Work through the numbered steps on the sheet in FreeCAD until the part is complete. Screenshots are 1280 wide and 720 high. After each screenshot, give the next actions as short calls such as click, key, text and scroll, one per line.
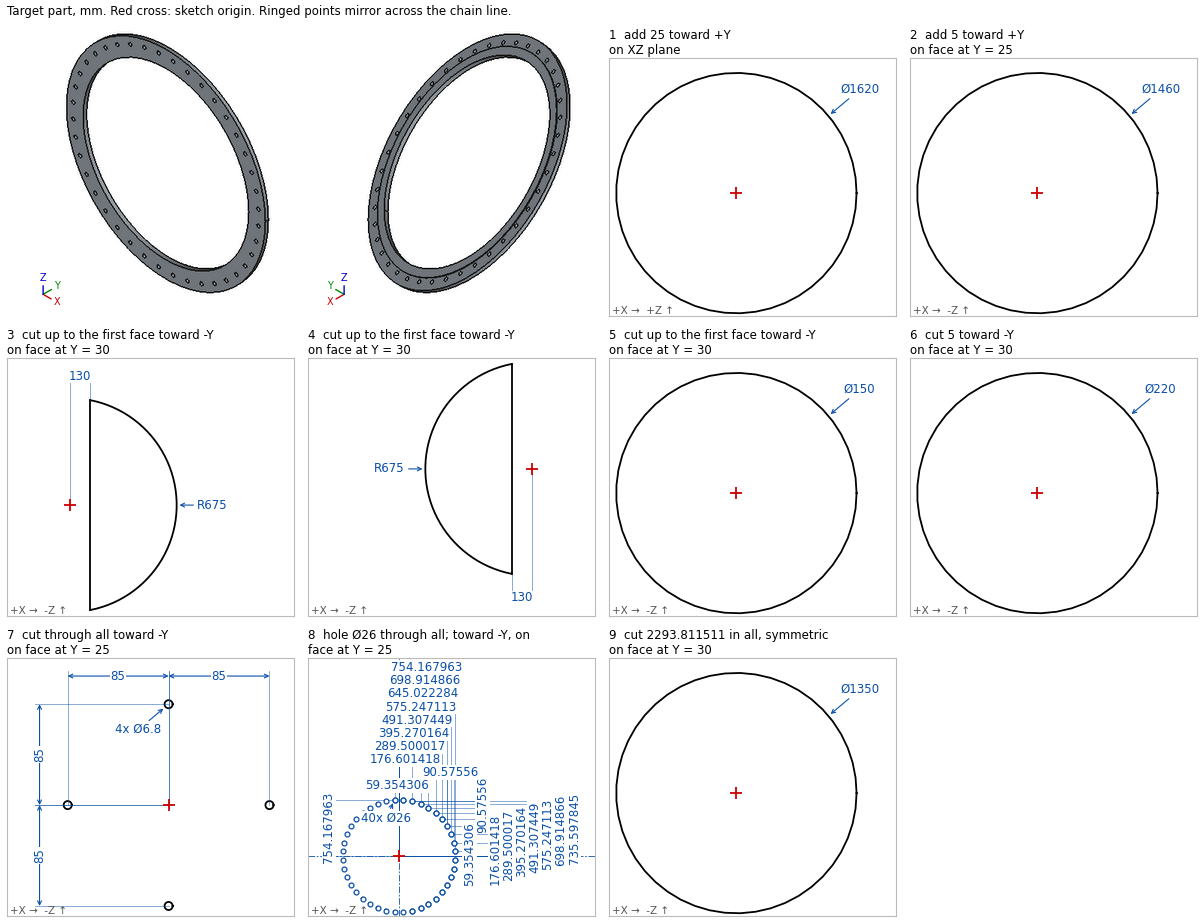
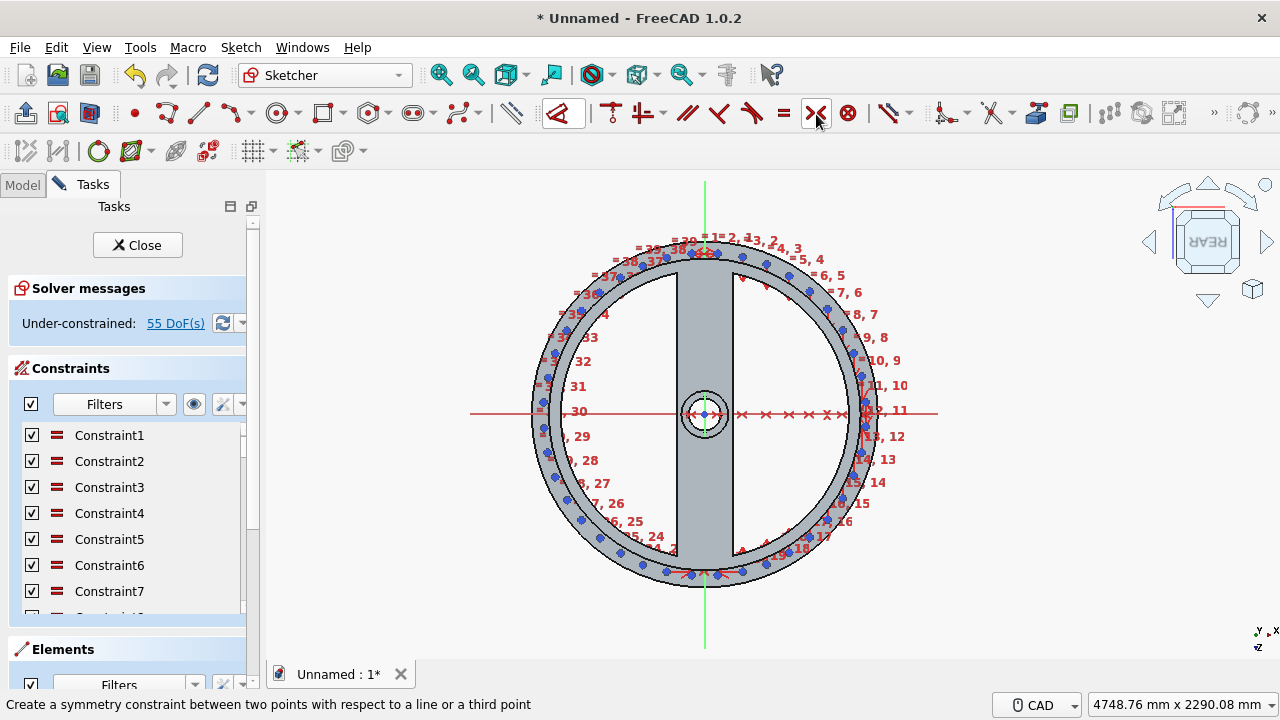
click(767, 565)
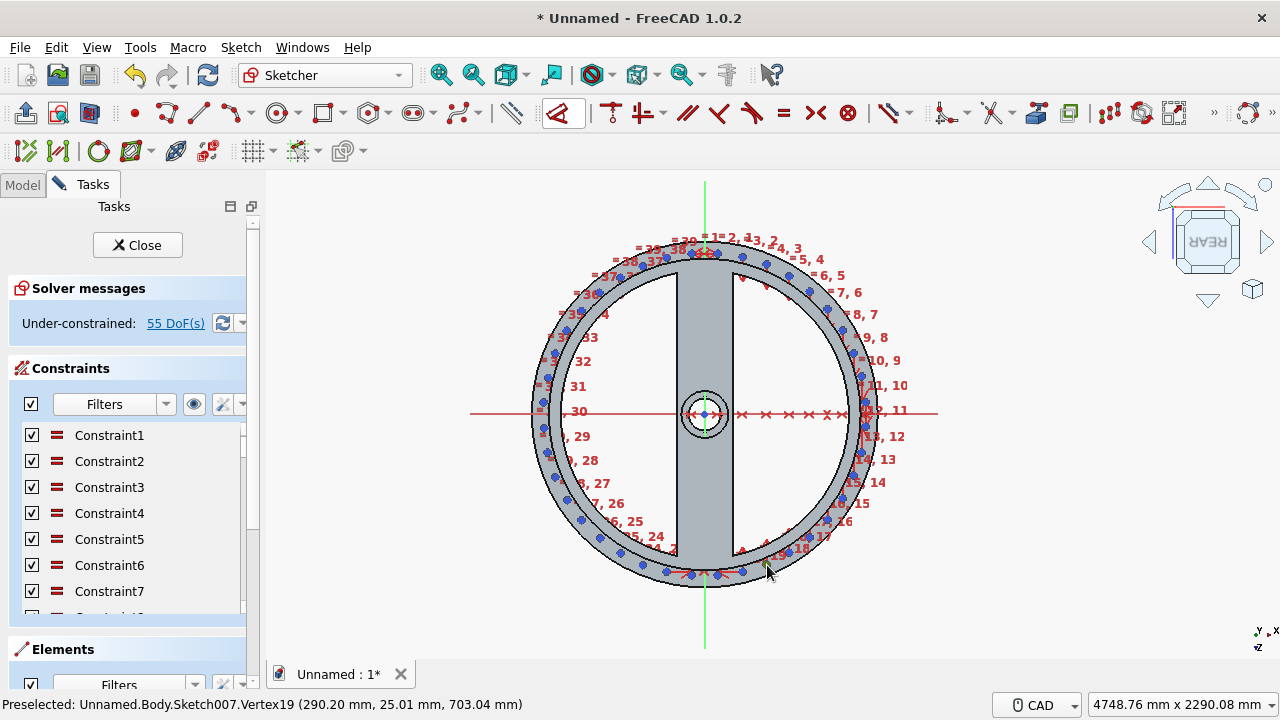
click(643, 565)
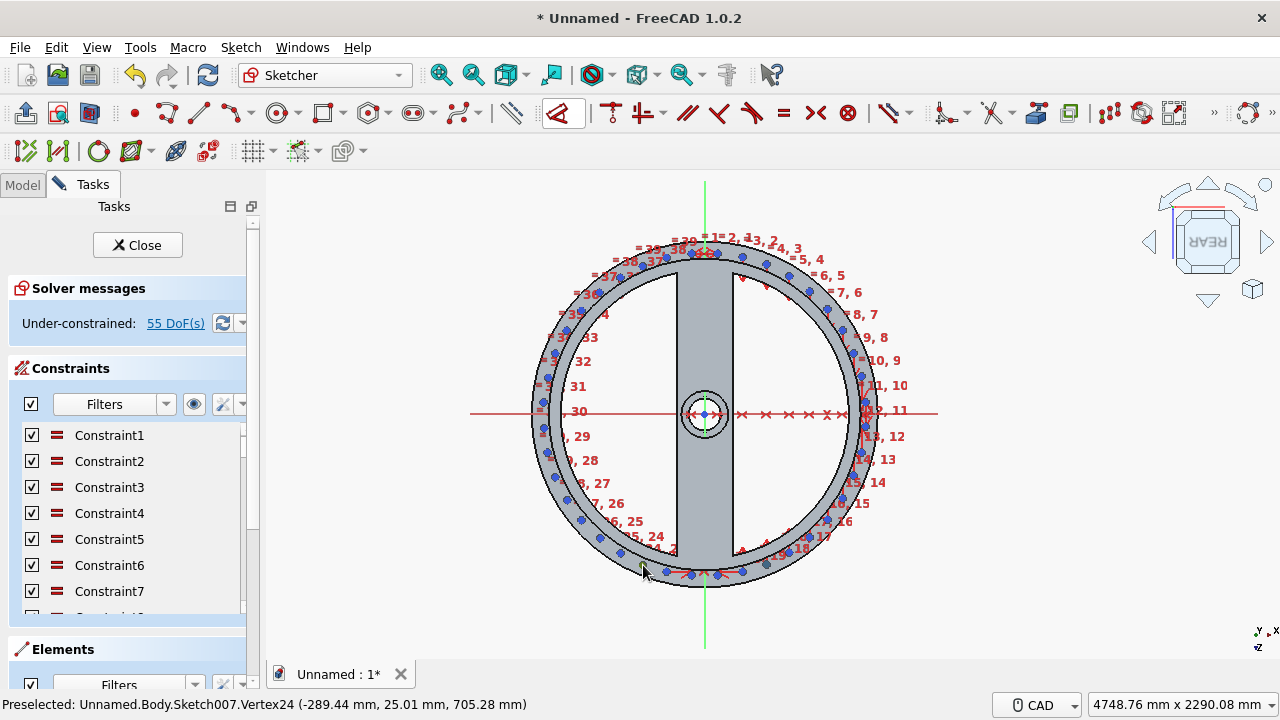
click(705, 538)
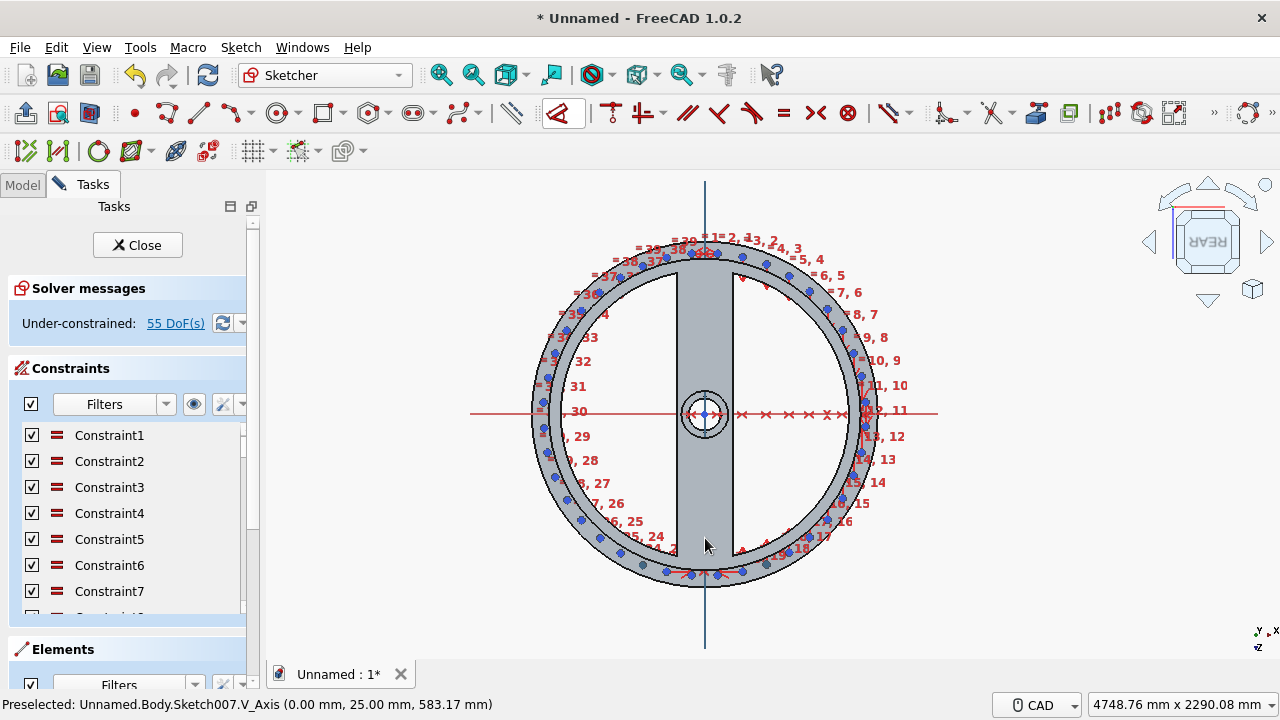
click(816, 114)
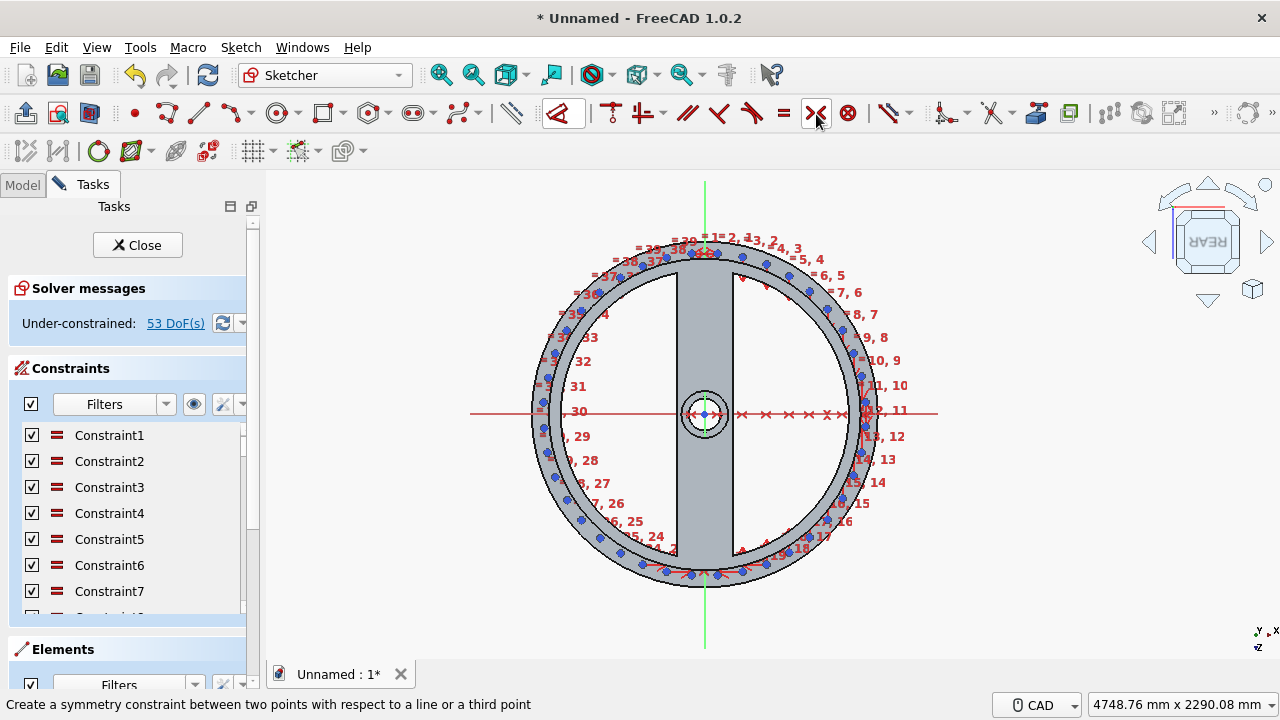
click(789, 553)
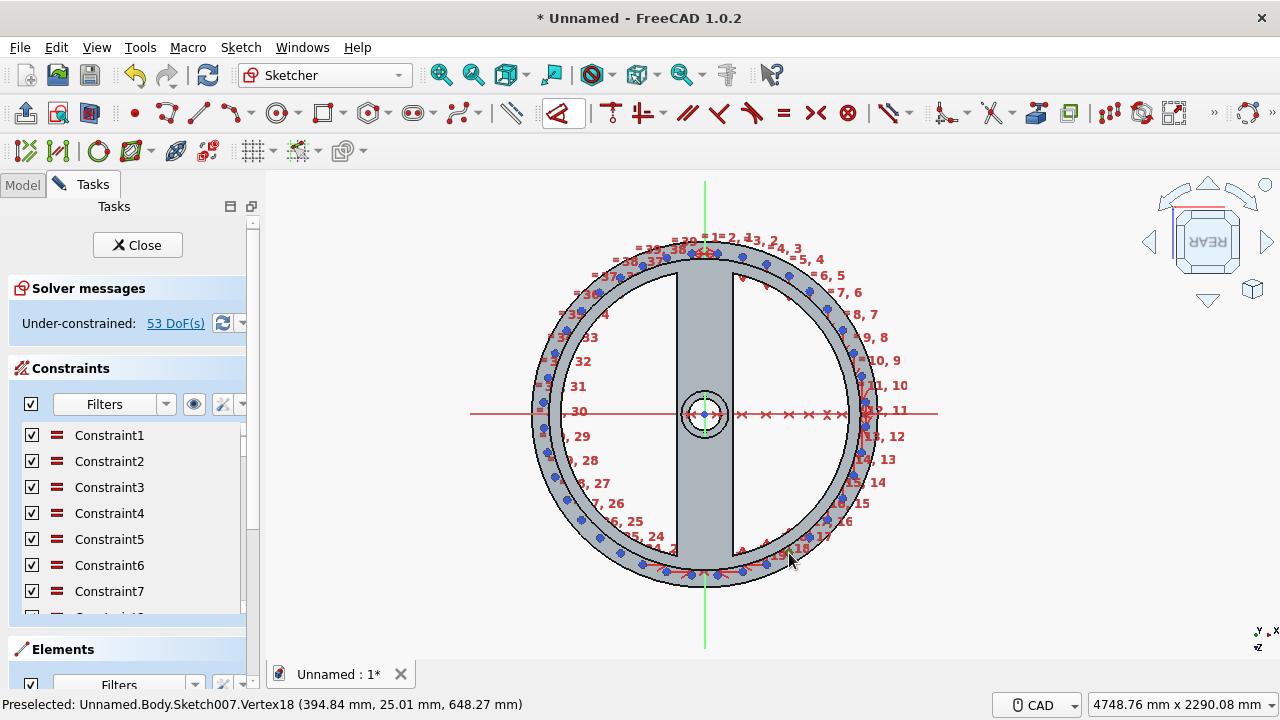
click(621, 553)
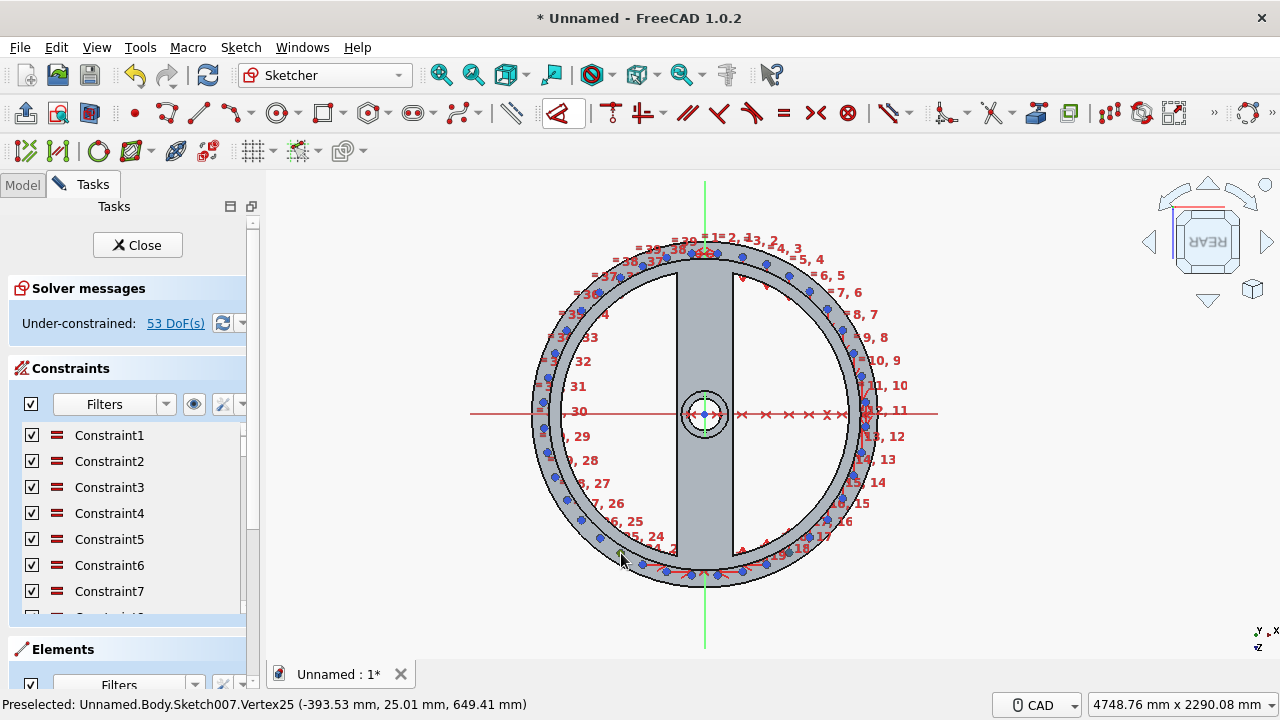
click(705, 538)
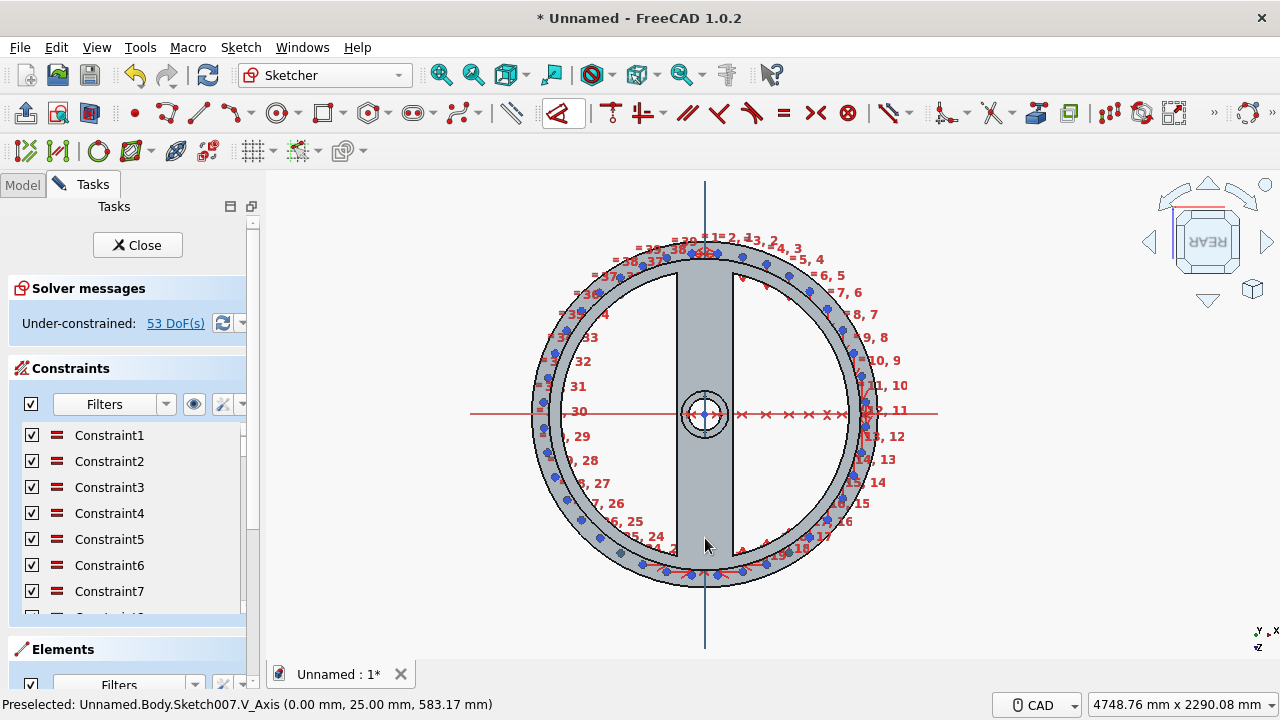
key(s)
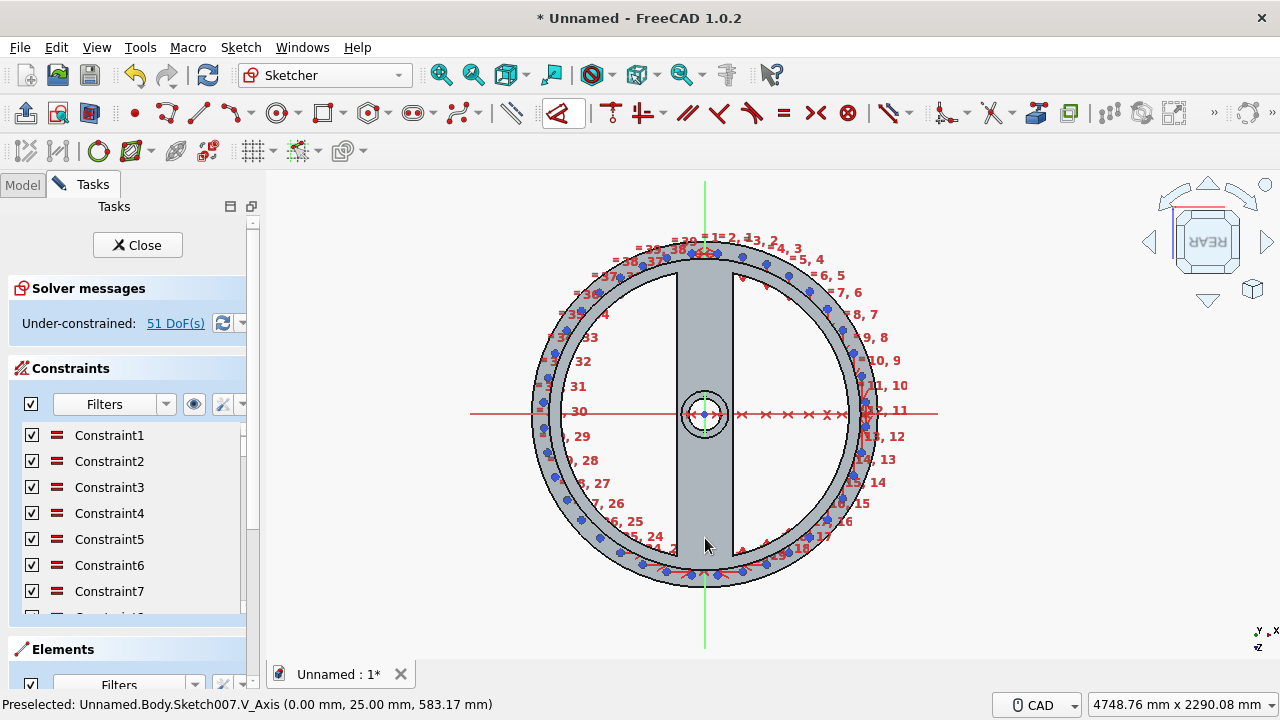
click(810, 537)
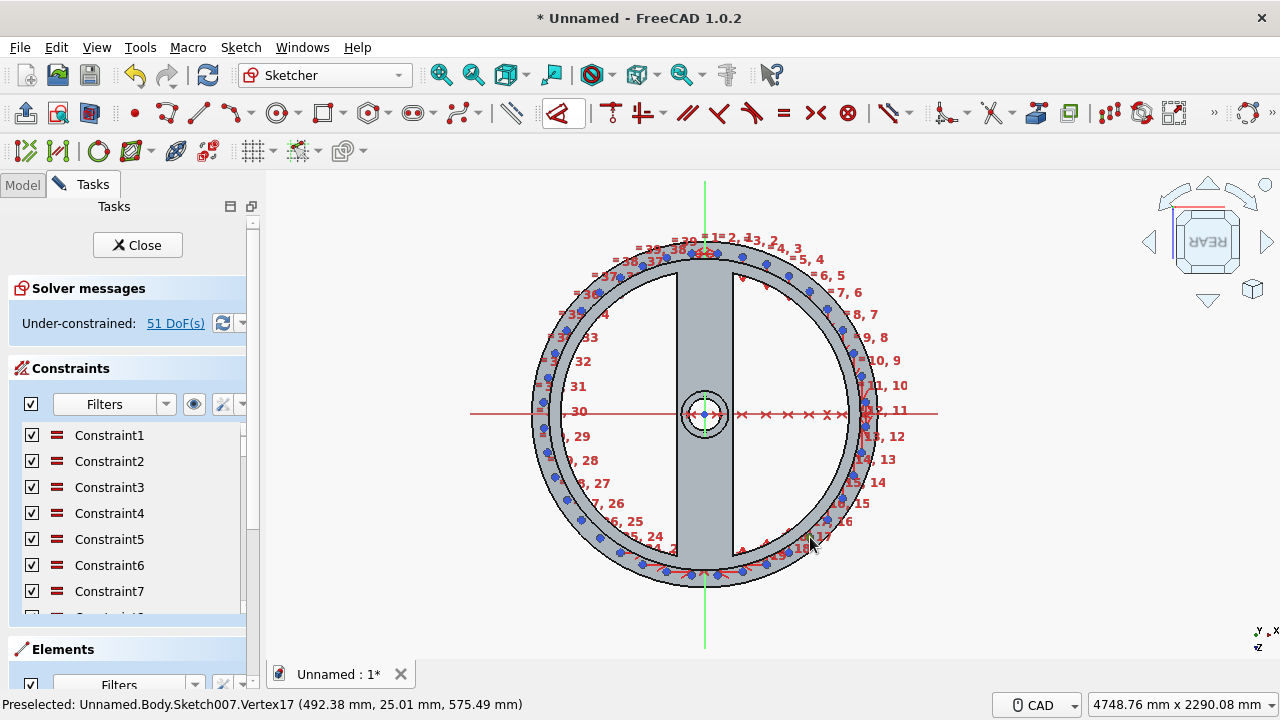
click(600, 538)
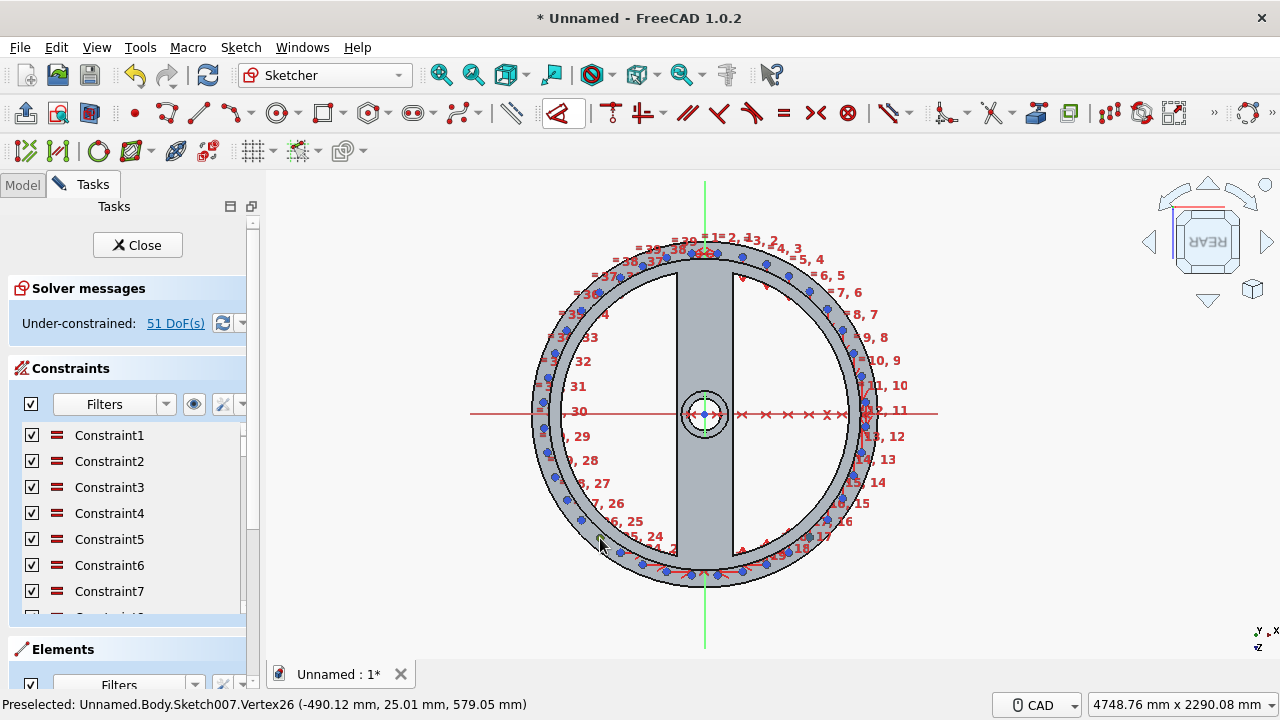
click(705, 538)